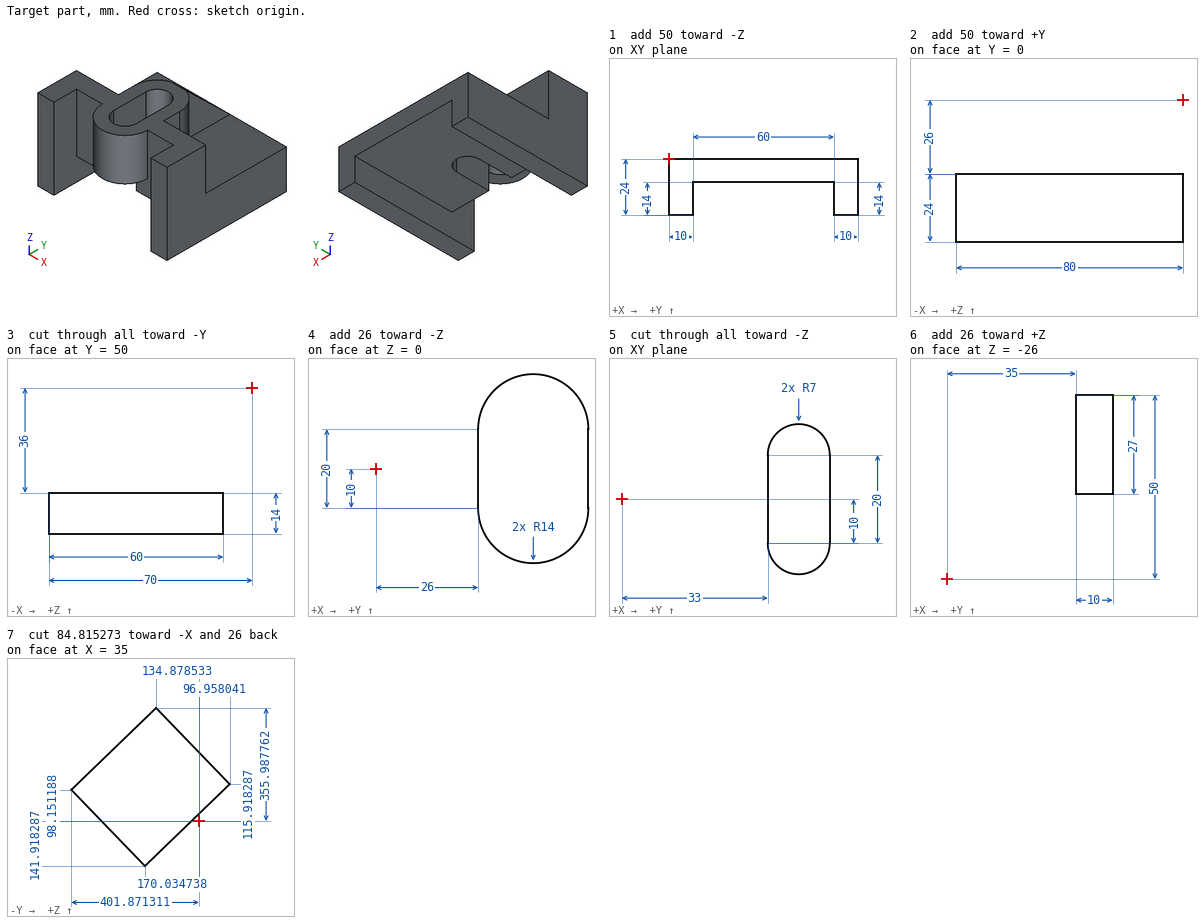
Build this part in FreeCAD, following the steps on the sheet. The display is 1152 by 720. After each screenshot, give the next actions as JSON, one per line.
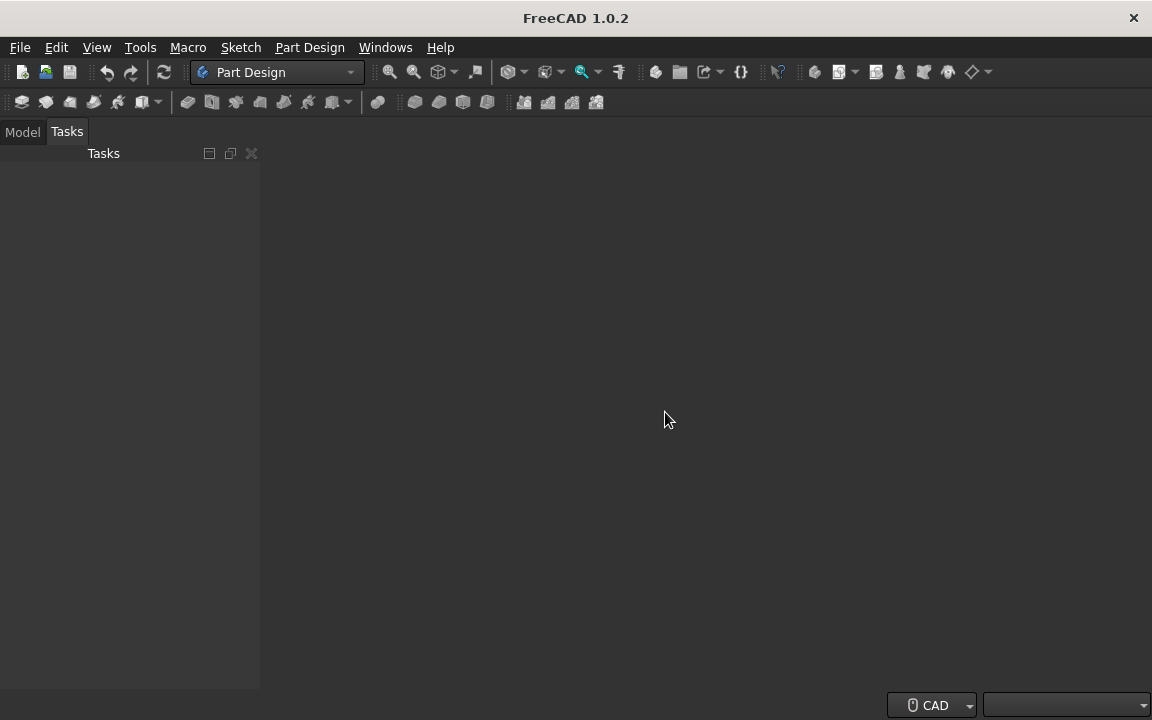
{"action": "key", "text": "ctrl+n"}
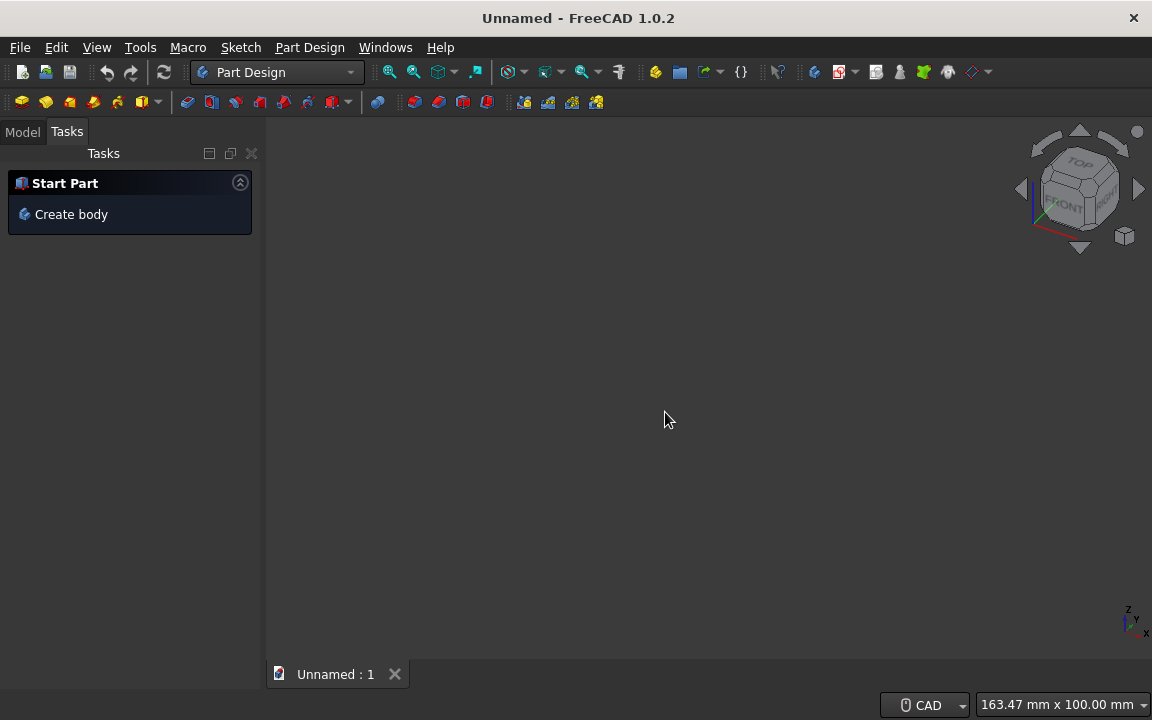
{"action": "left_click", "coordinate": [840, 72]}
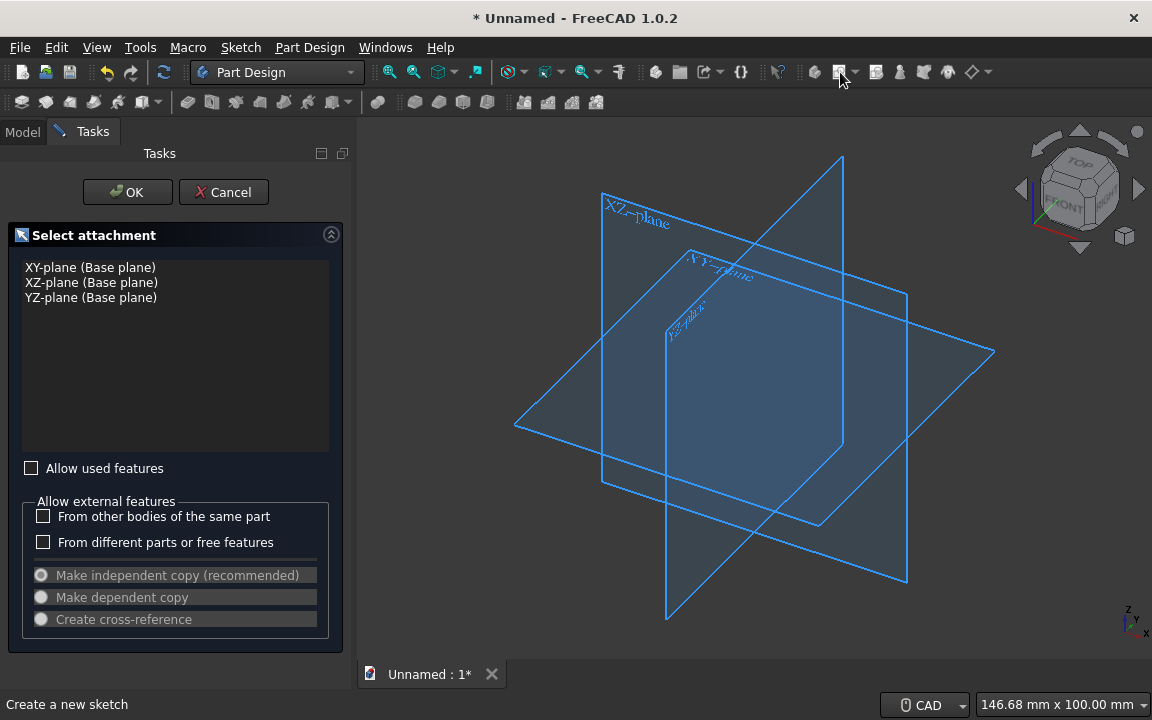
{"action": "left_click", "coordinate": [82, 268]}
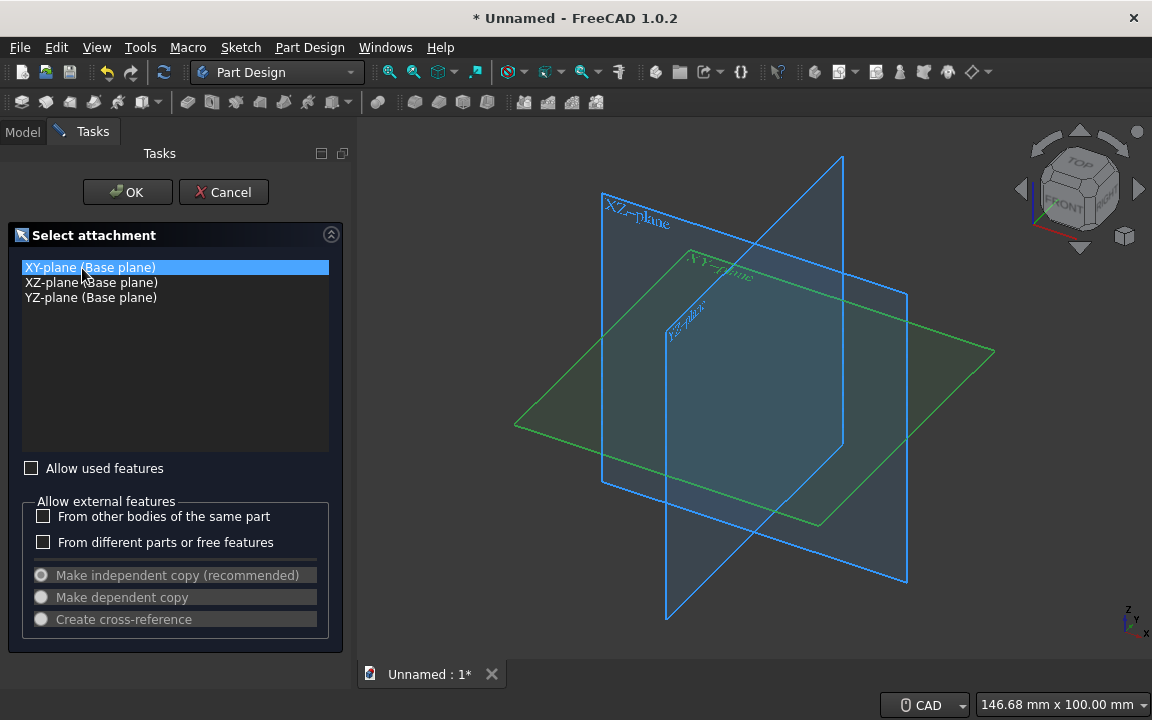
{"action": "left_click", "coordinate": [128, 192]}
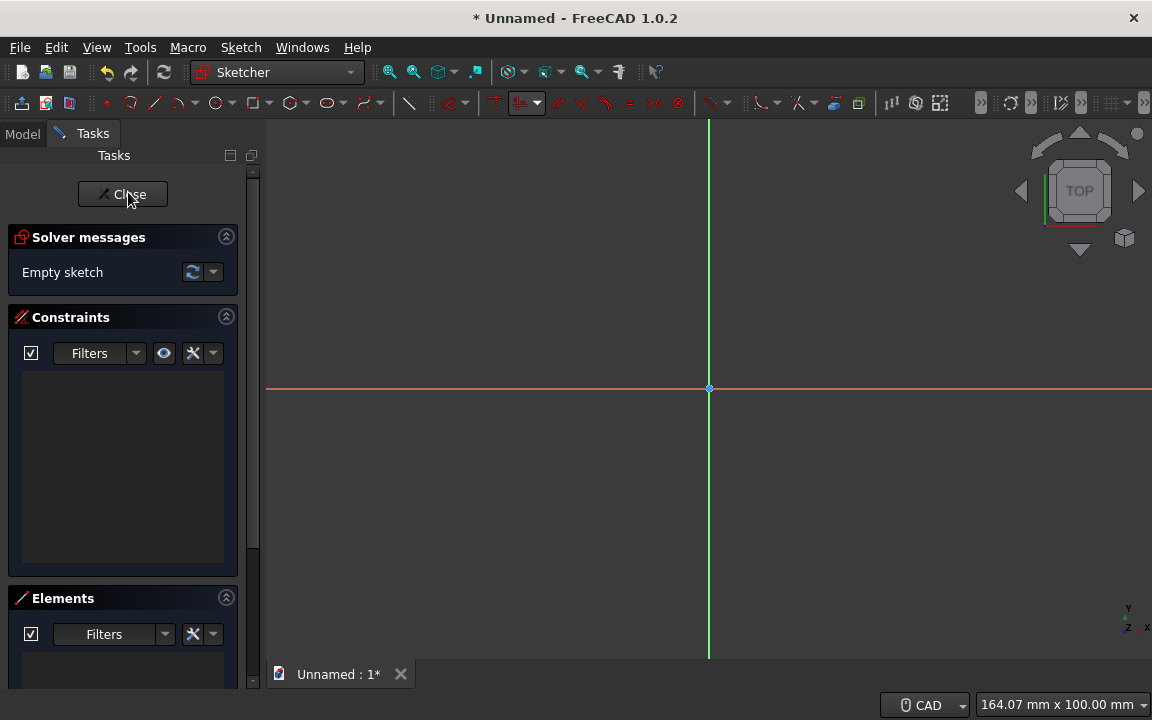
{"action": "scroll", "coordinate": [294, 257], "scroll_direction": "down", "scroll_amount": 2}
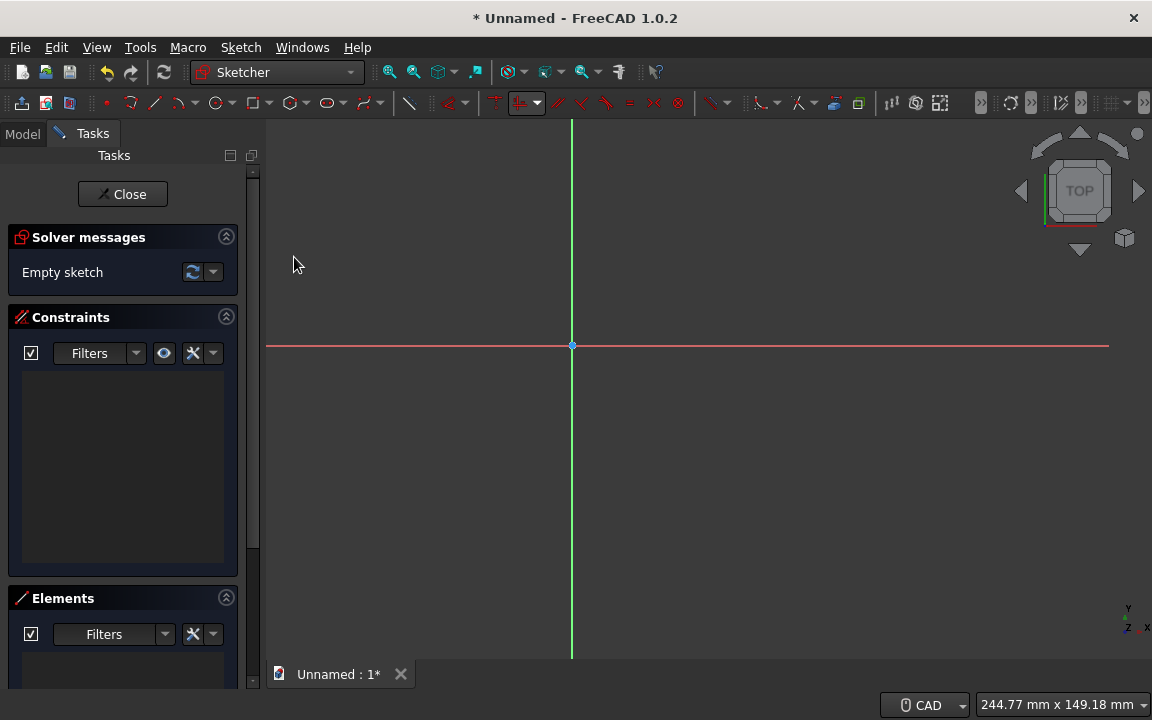
{"action": "scroll", "coordinate": [810, 389], "scroll_direction": "up", "scroll_amount": 3}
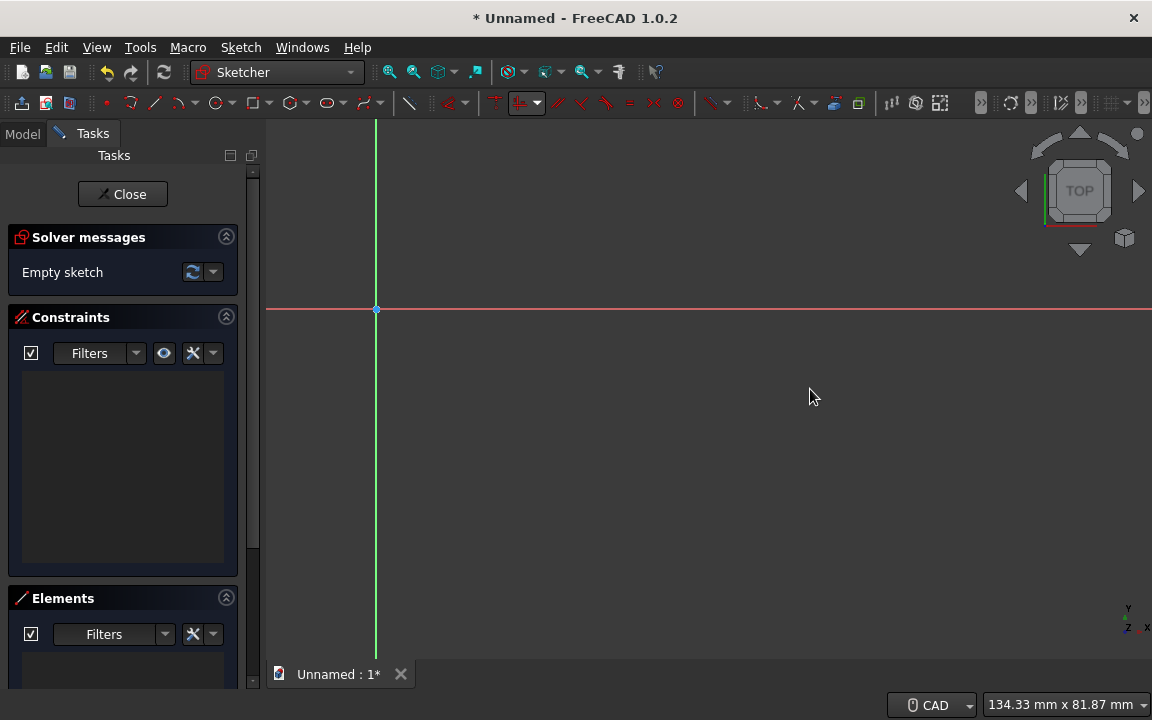
{"action": "key", "text": "g m"}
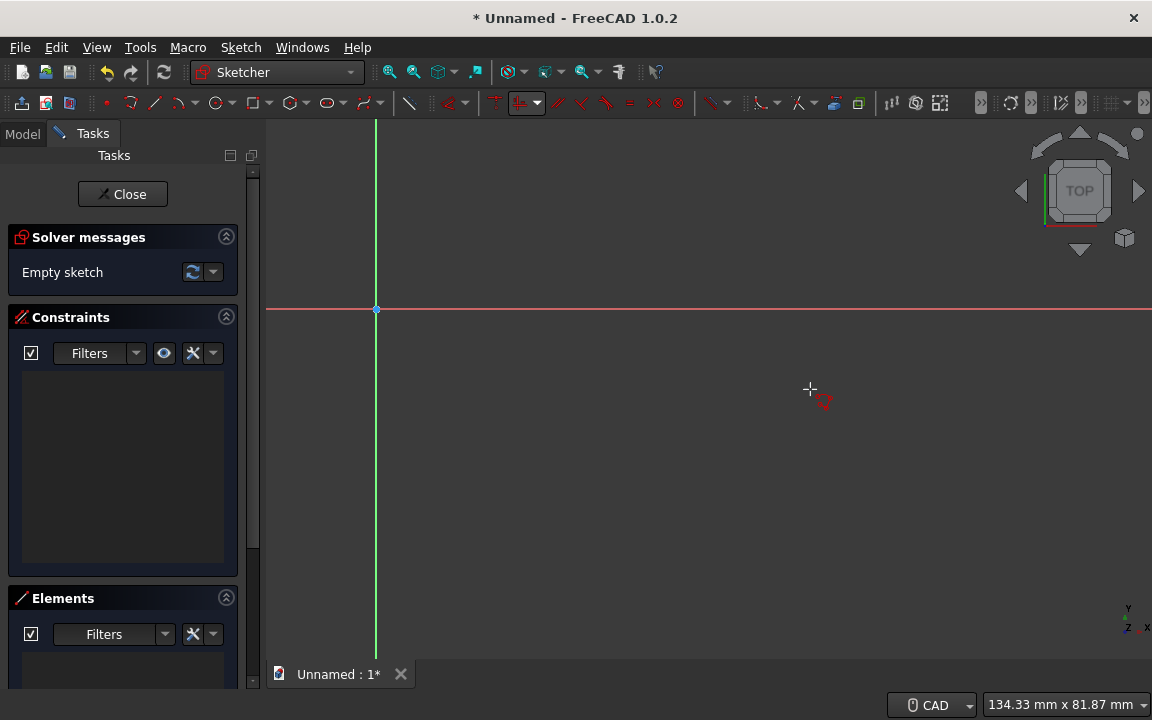
{"action": "left_click", "coordinate": [376, 309]}
{"action": "left_click", "coordinate": [385, 468]}
{"action": "left_click", "coordinate": [442, 468]}
{"action": "left_click", "coordinate": [442, 375]}
{"action": "left_click", "coordinate": [838, 375]}
{"action": "left_click", "coordinate": [838, 468]}
{"action": "left_click", "coordinate": [904, 468]}
{"action": "left_click", "coordinate": [904, 318]}
{"action": "left_click", "coordinate": [376, 309]}
{"action": "key", "text": "Escape"}
{"action": "key", "text": "Escape"}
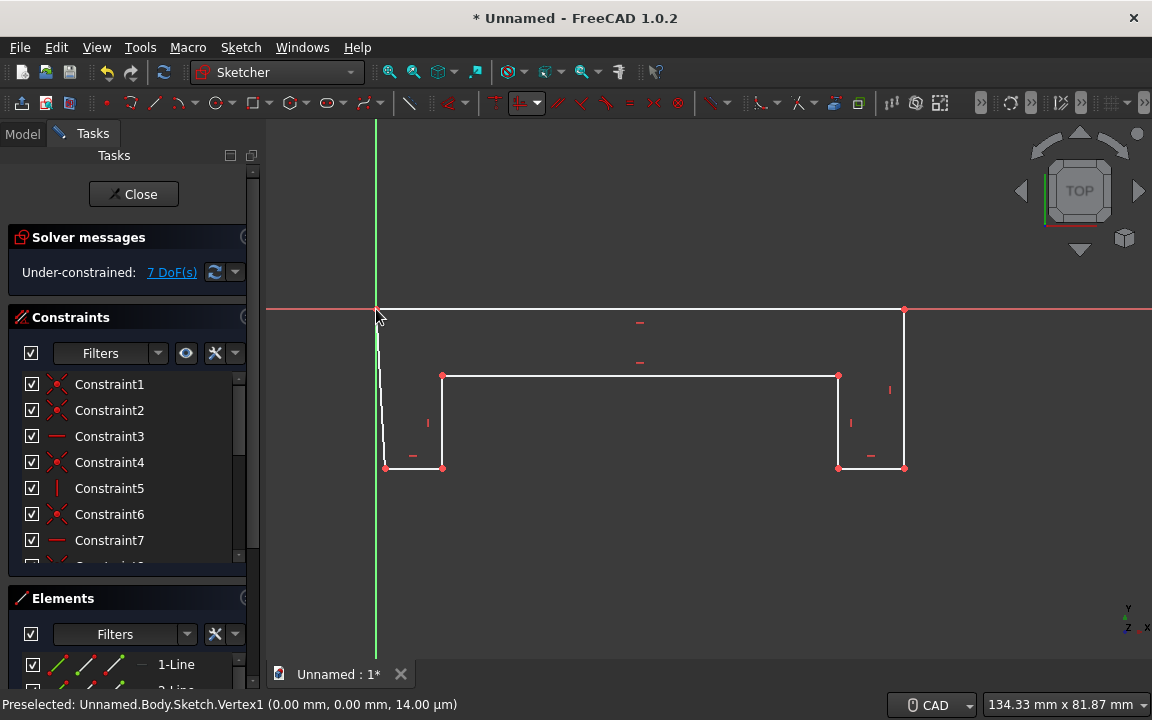
{"action": "left_click", "coordinate": [379, 357]}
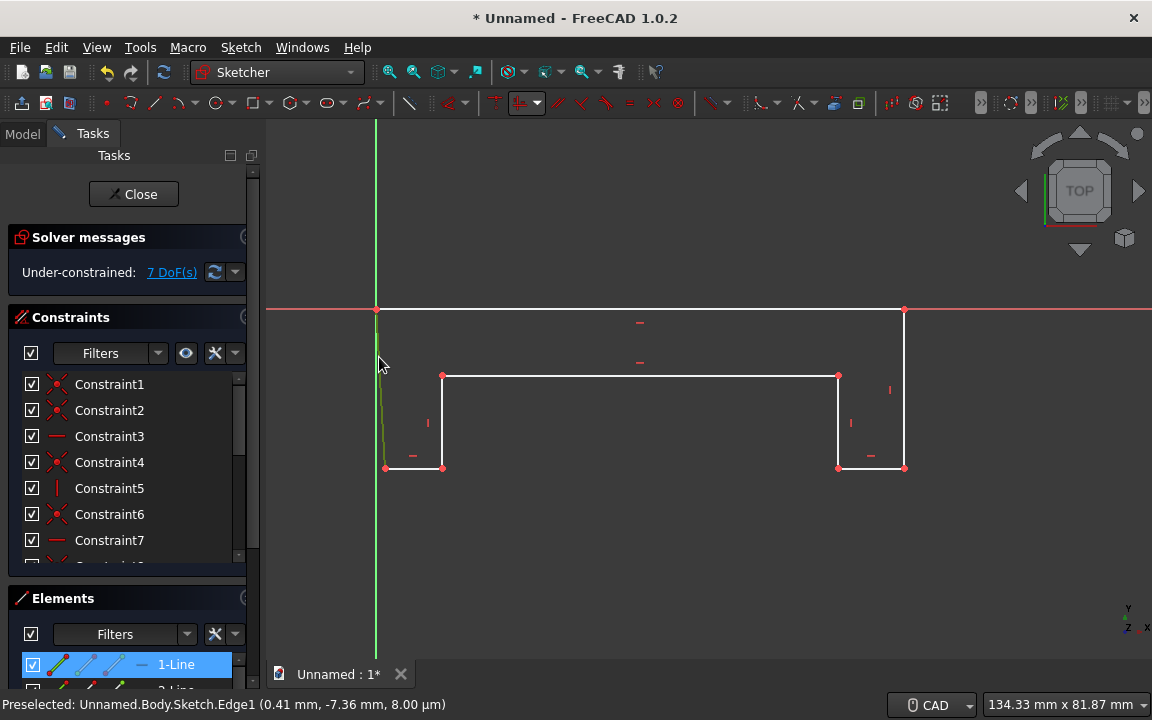
{"action": "left_click", "coordinate": [540, 104]}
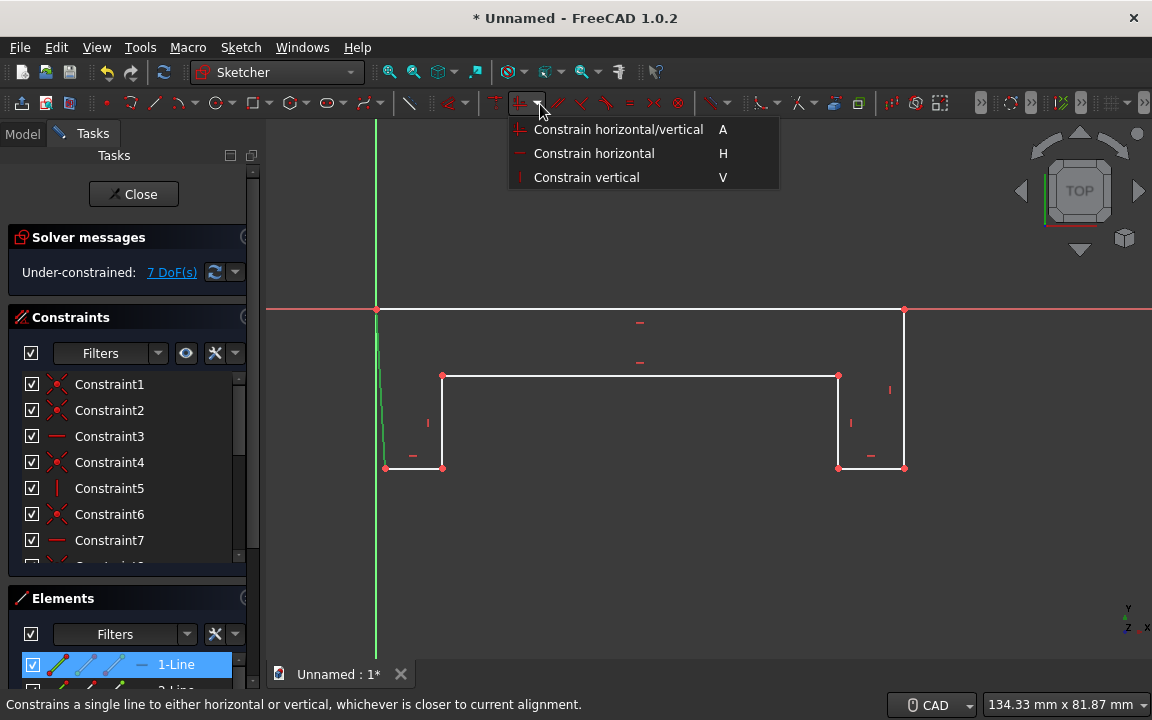
{"action": "left_click", "coordinate": [644, 177]}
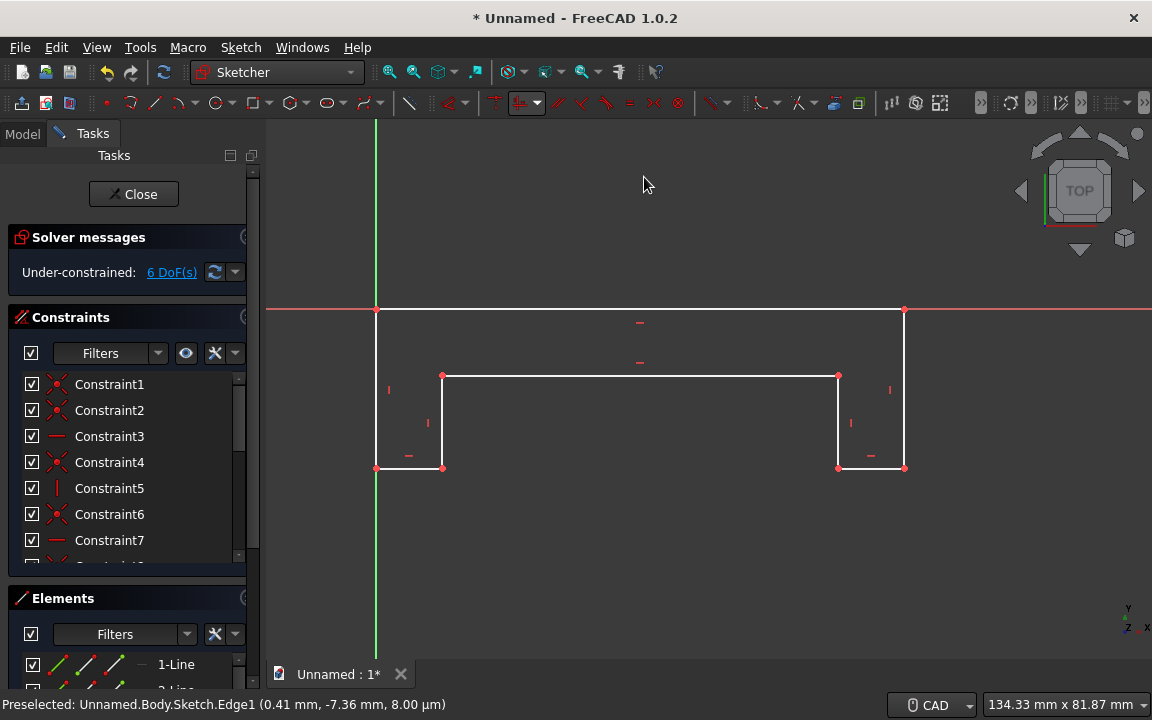
{"action": "left_click", "coordinate": [448, 104]}